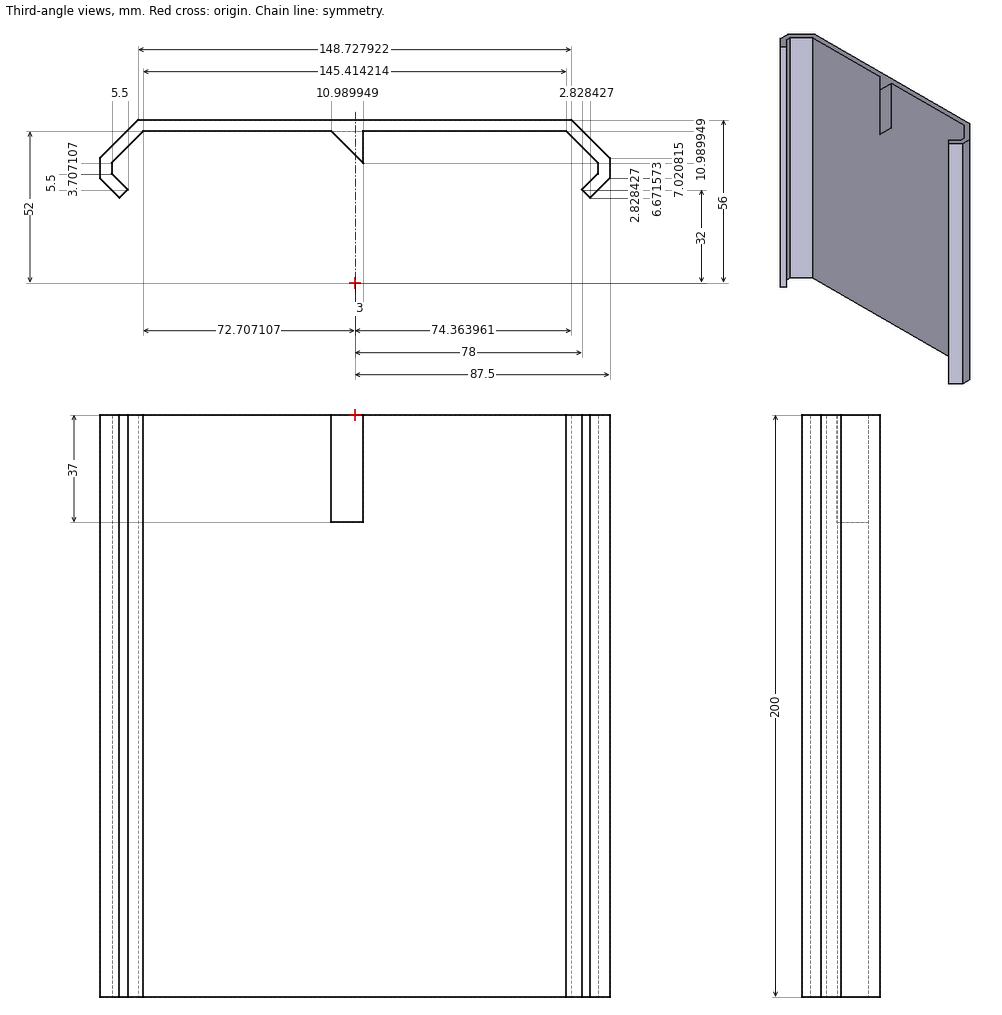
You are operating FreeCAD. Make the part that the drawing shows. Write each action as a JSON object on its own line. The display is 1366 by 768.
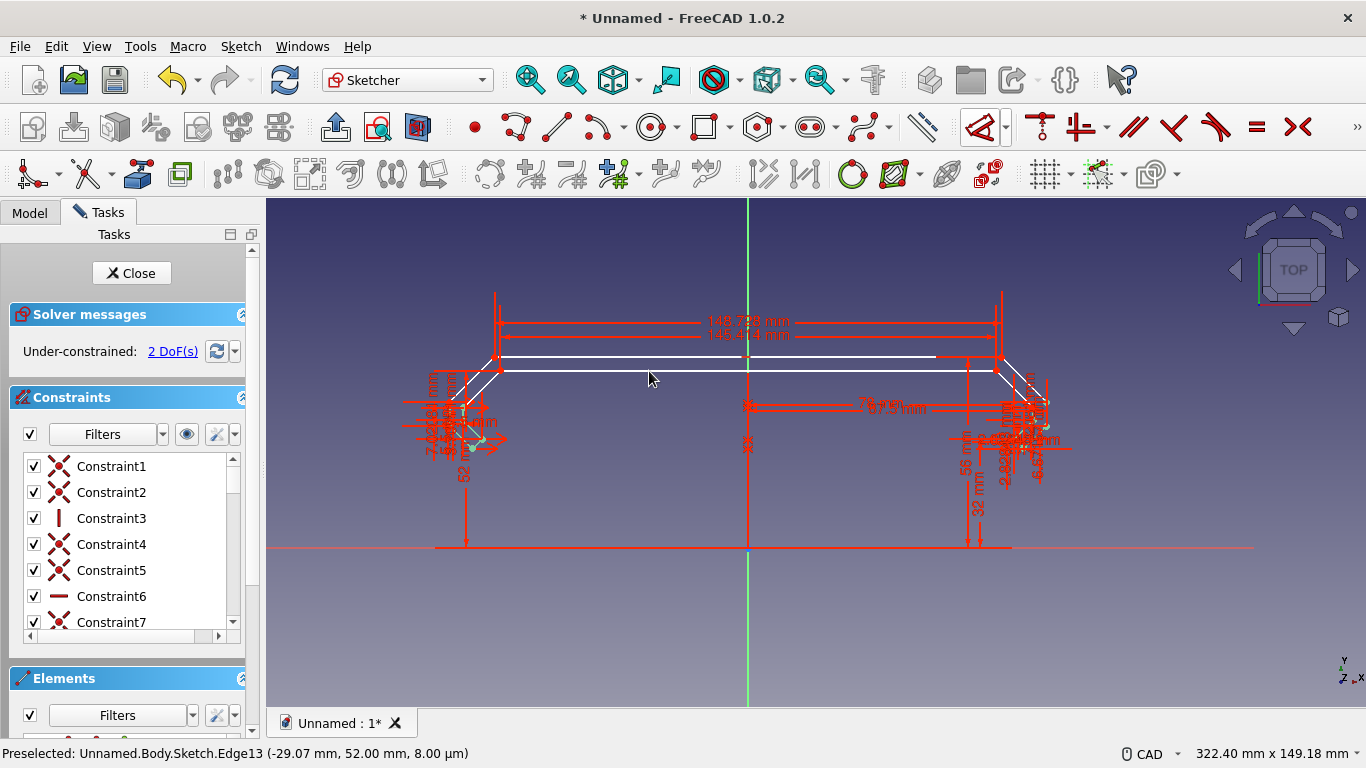
{"action": "left_click", "coordinate": [1002, 357]}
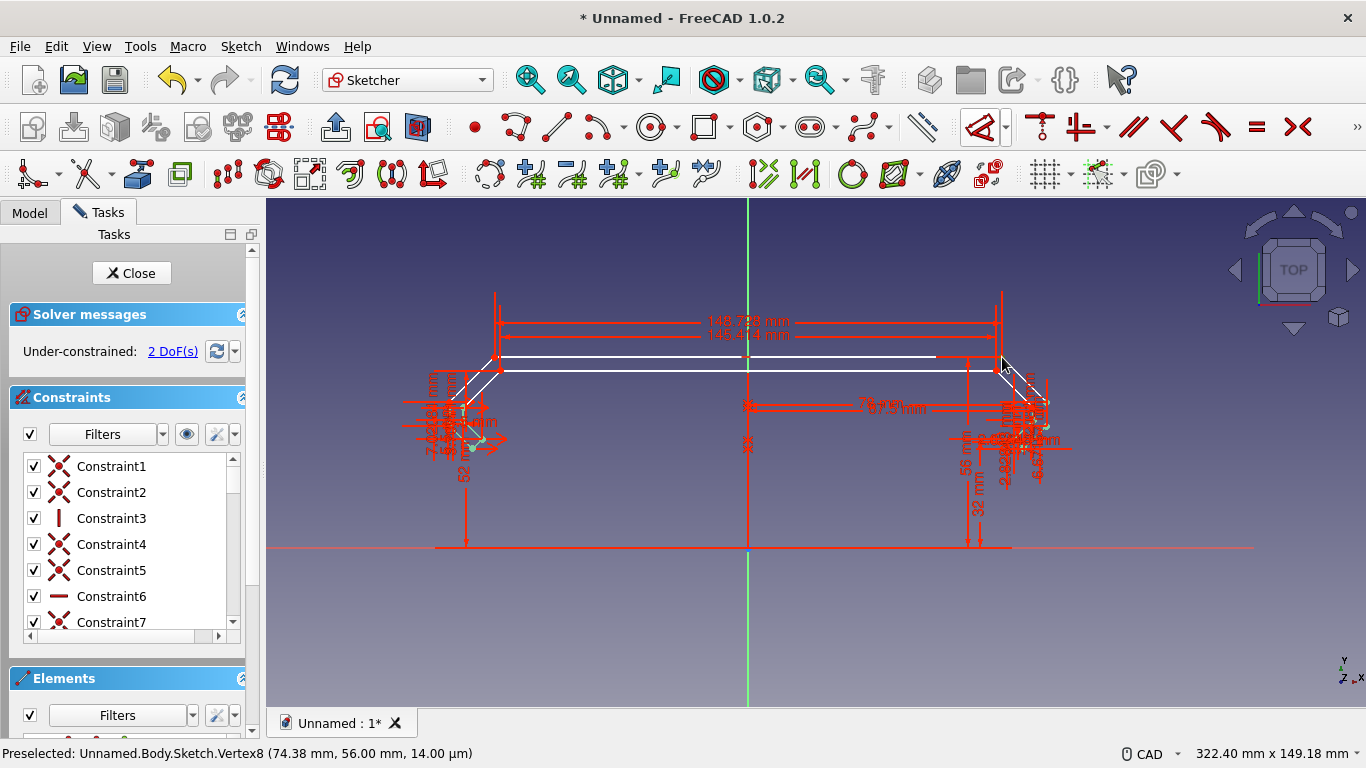
{"action": "left_click", "coordinate": [1006, 128]}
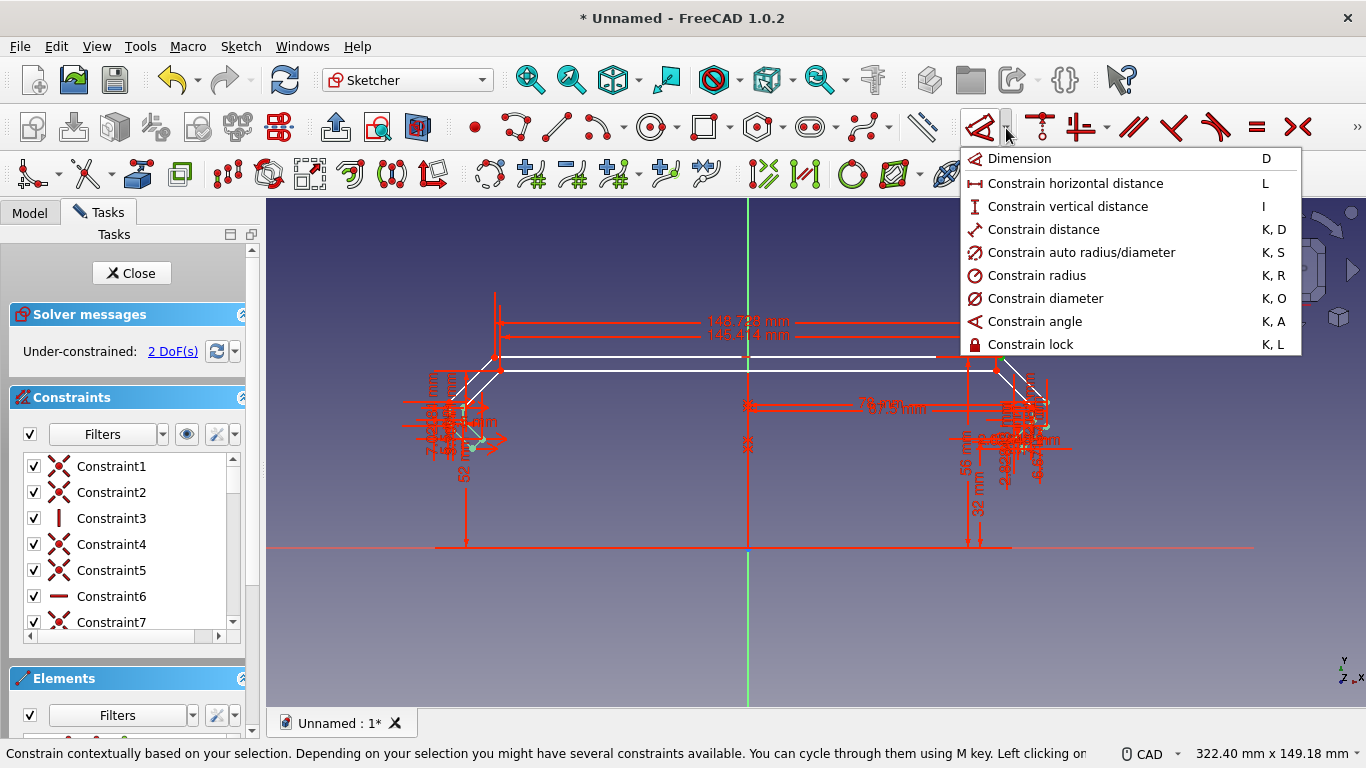
{"action": "left_click", "coordinate": [1131, 184]}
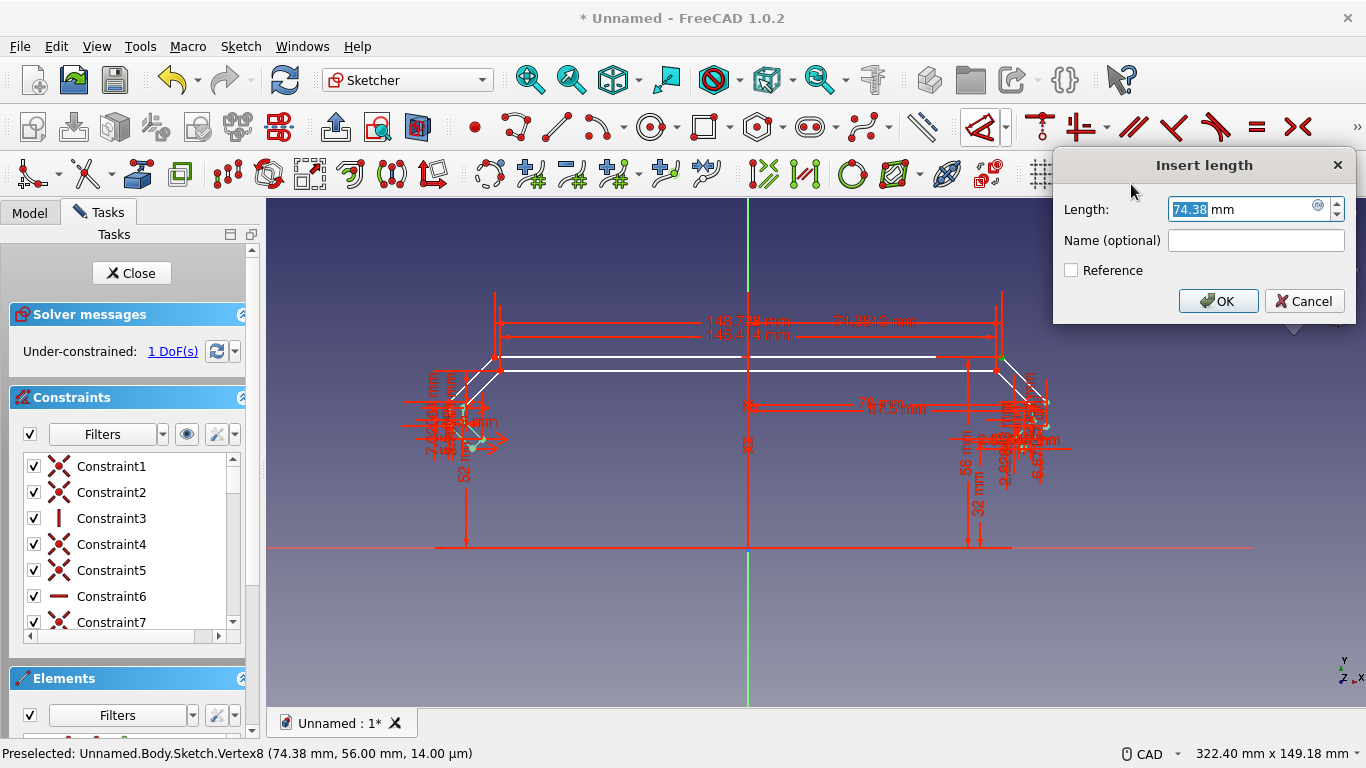
{"action": "type", "text": "74.363961"}
{"action": "key", "text": "Return"}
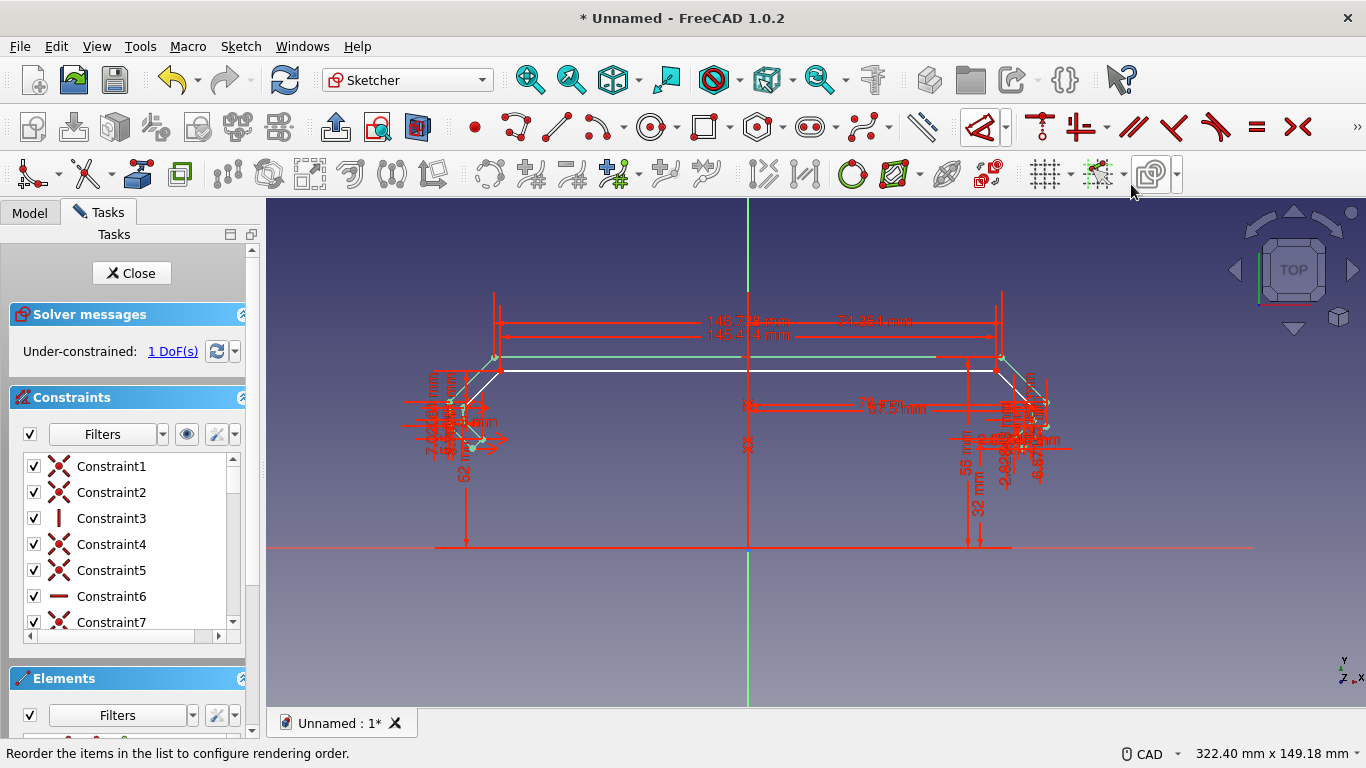
{"action": "left_click", "coordinate": [500, 371]}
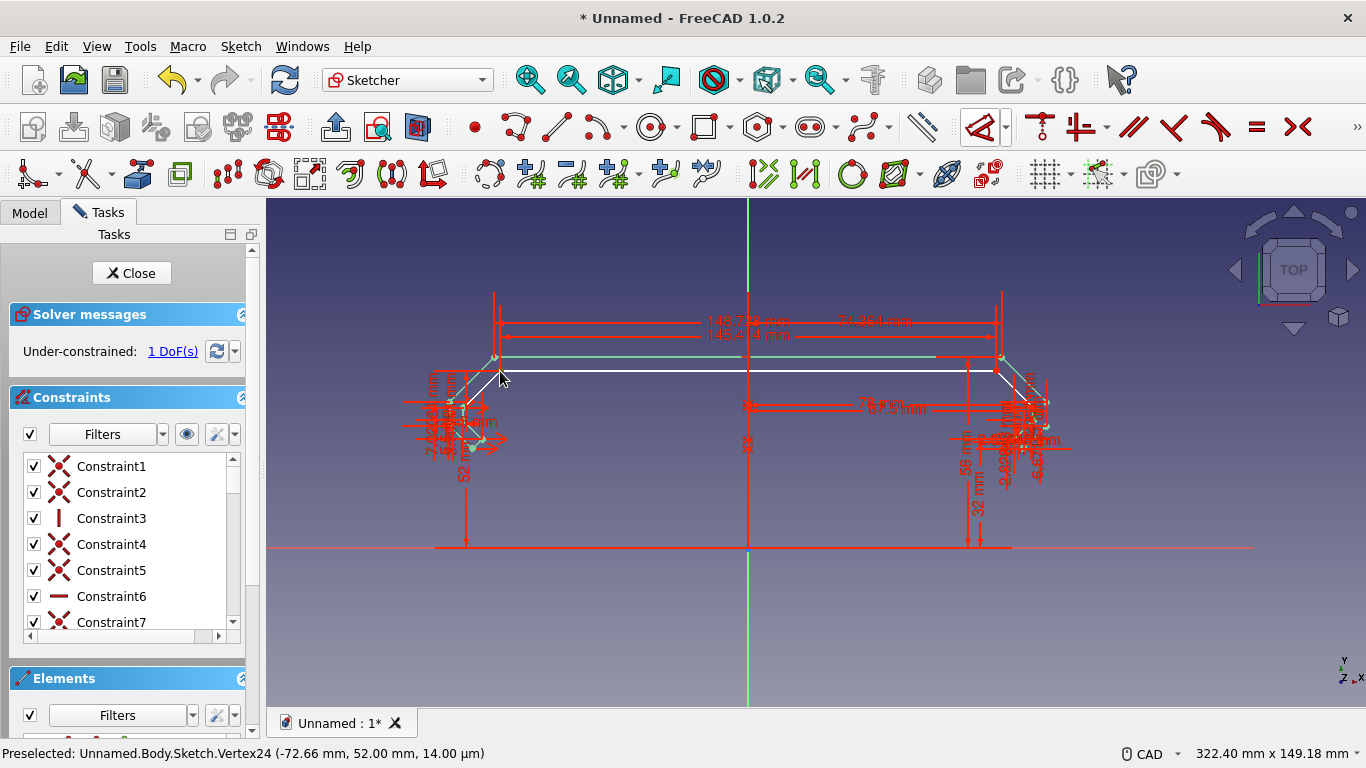
{"action": "left_click", "coordinate": [1006, 128]}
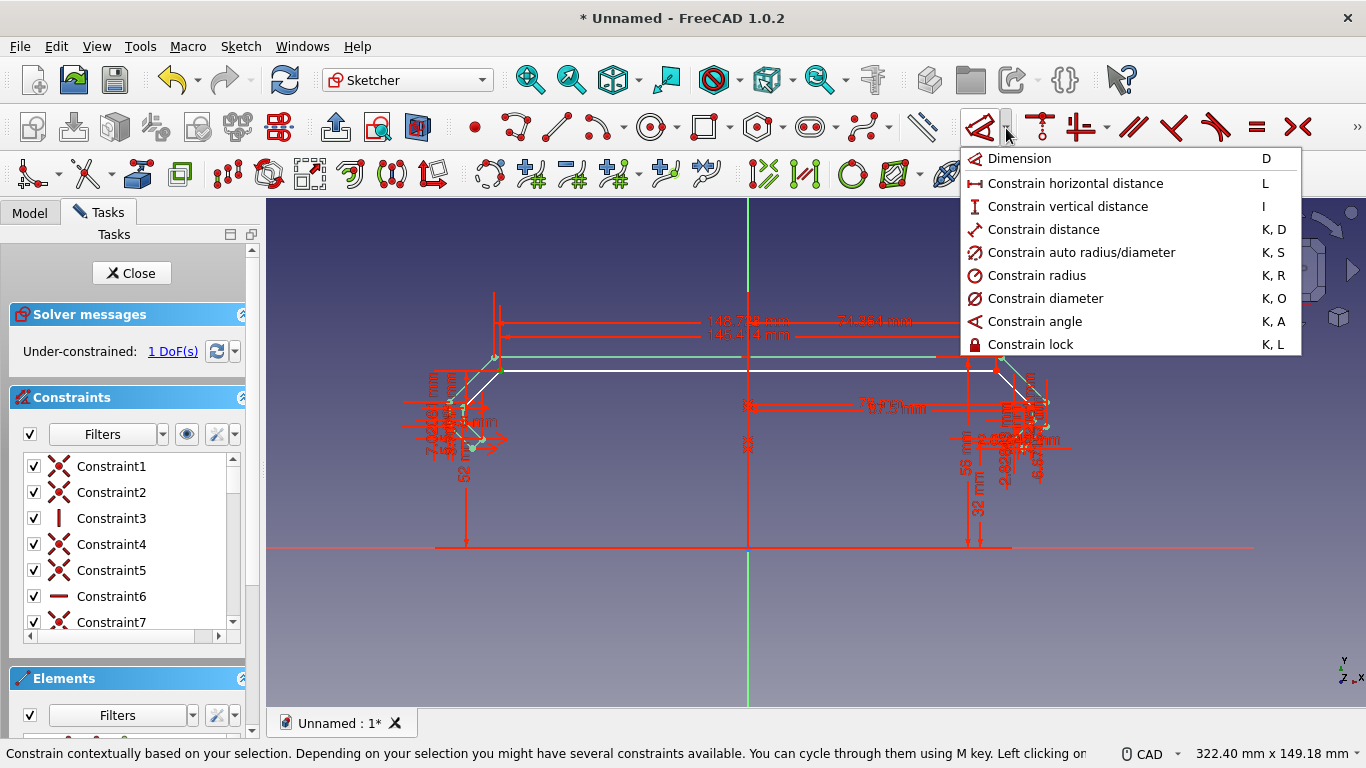
{"action": "left_click", "coordinate": [1131, 184]}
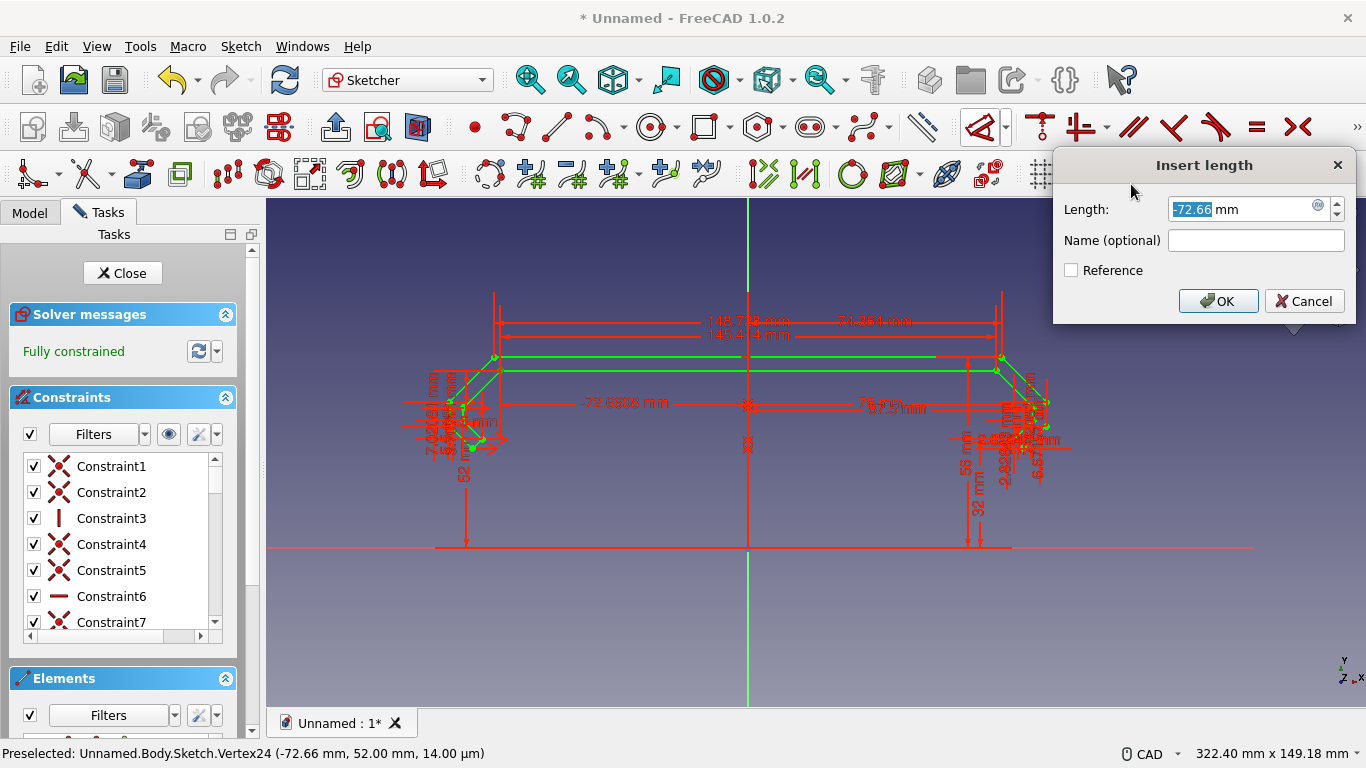
{"action": "type", "text": "-72.707107"}
{"action": "key", "text": "Return"}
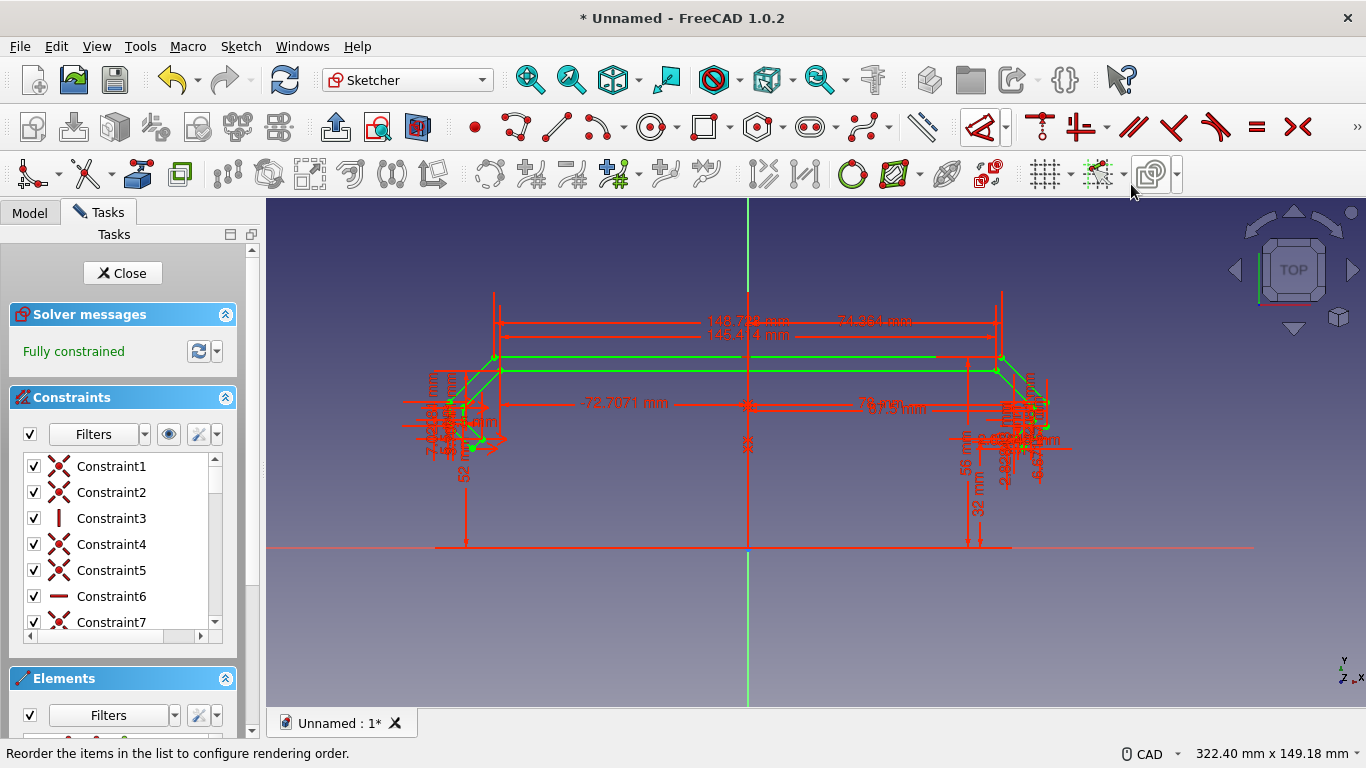
{"action": "left_click", "coordinate": [123, 273]}